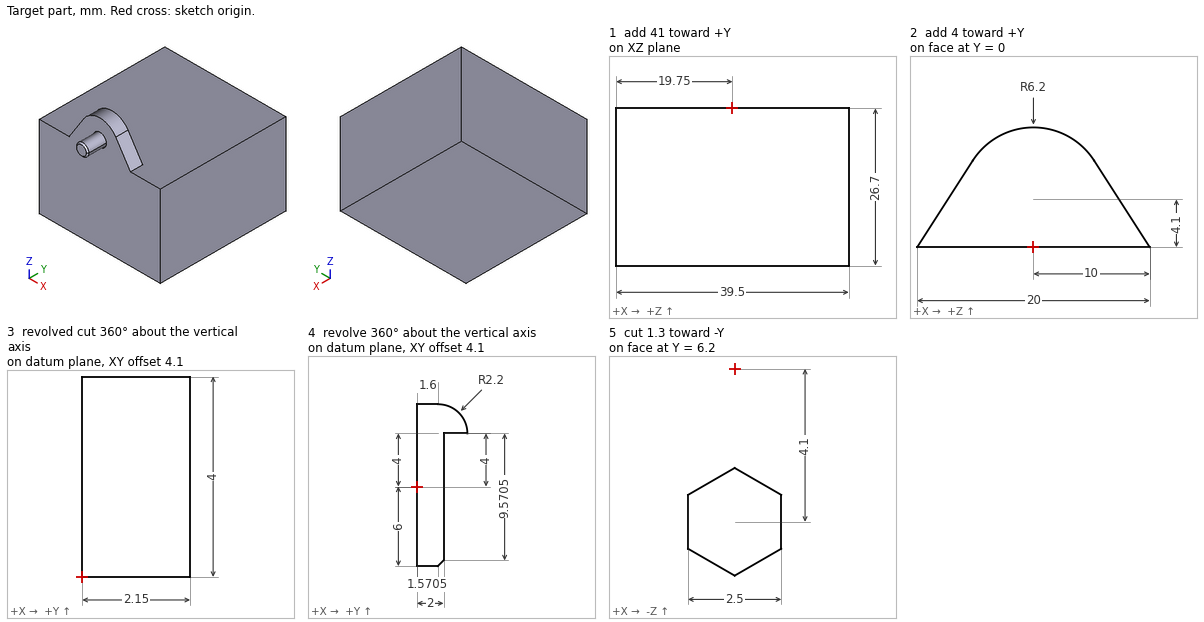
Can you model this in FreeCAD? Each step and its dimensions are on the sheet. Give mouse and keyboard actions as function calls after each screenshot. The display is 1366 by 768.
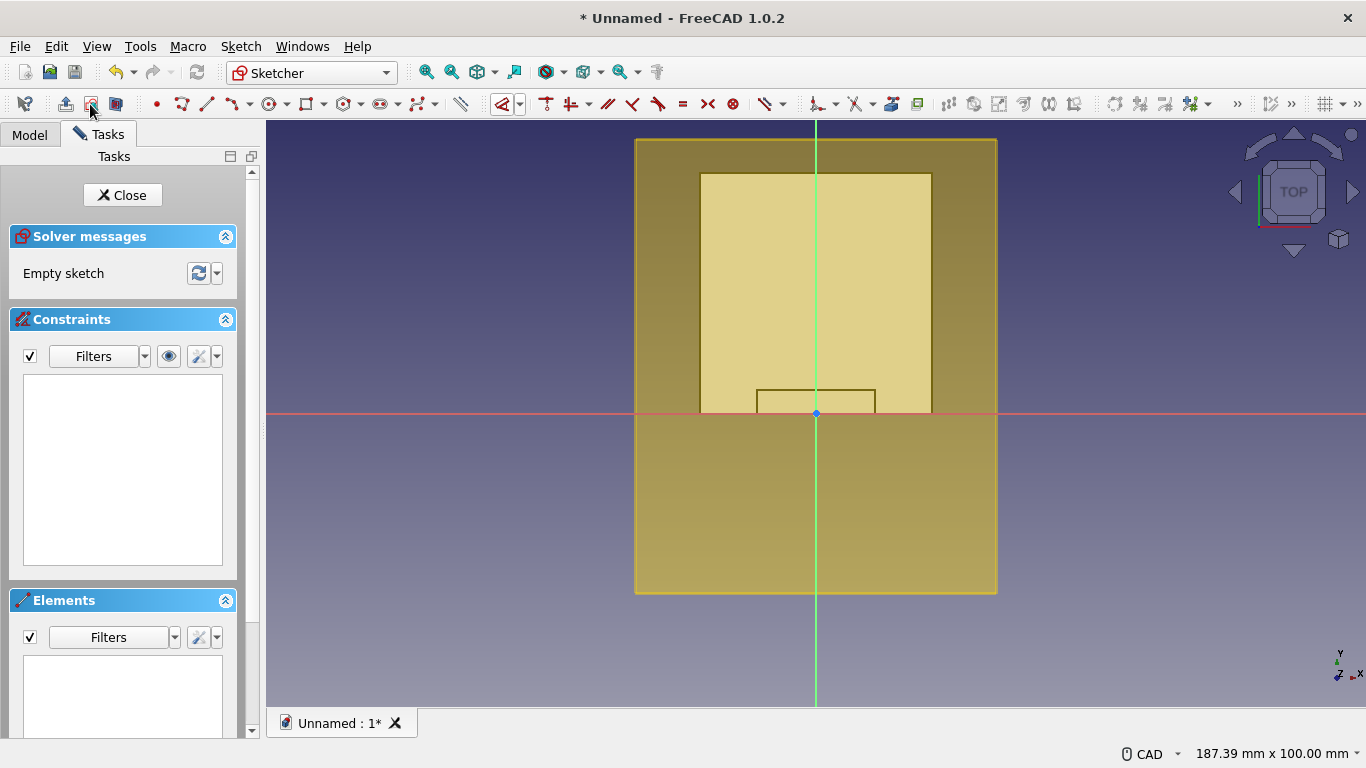
scroll(827, 401, up, 14)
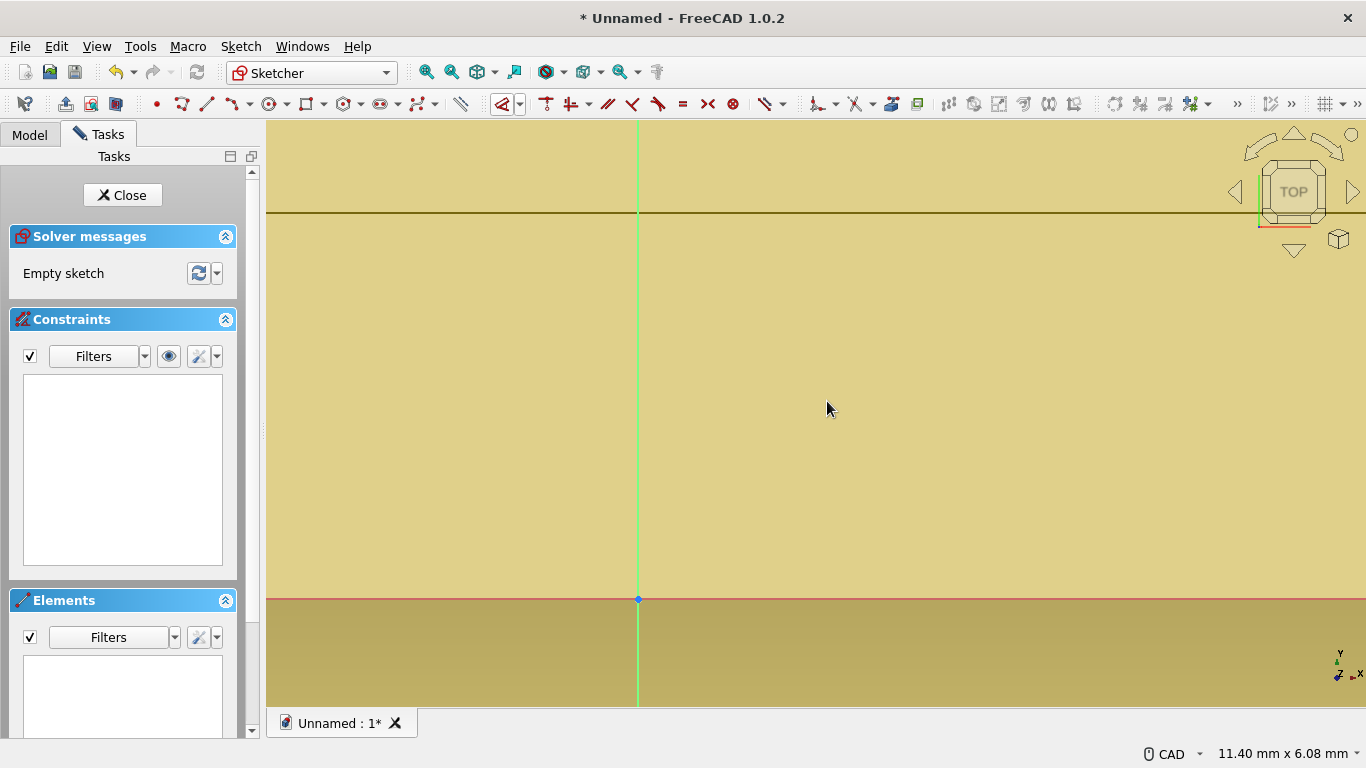
click(306, 104)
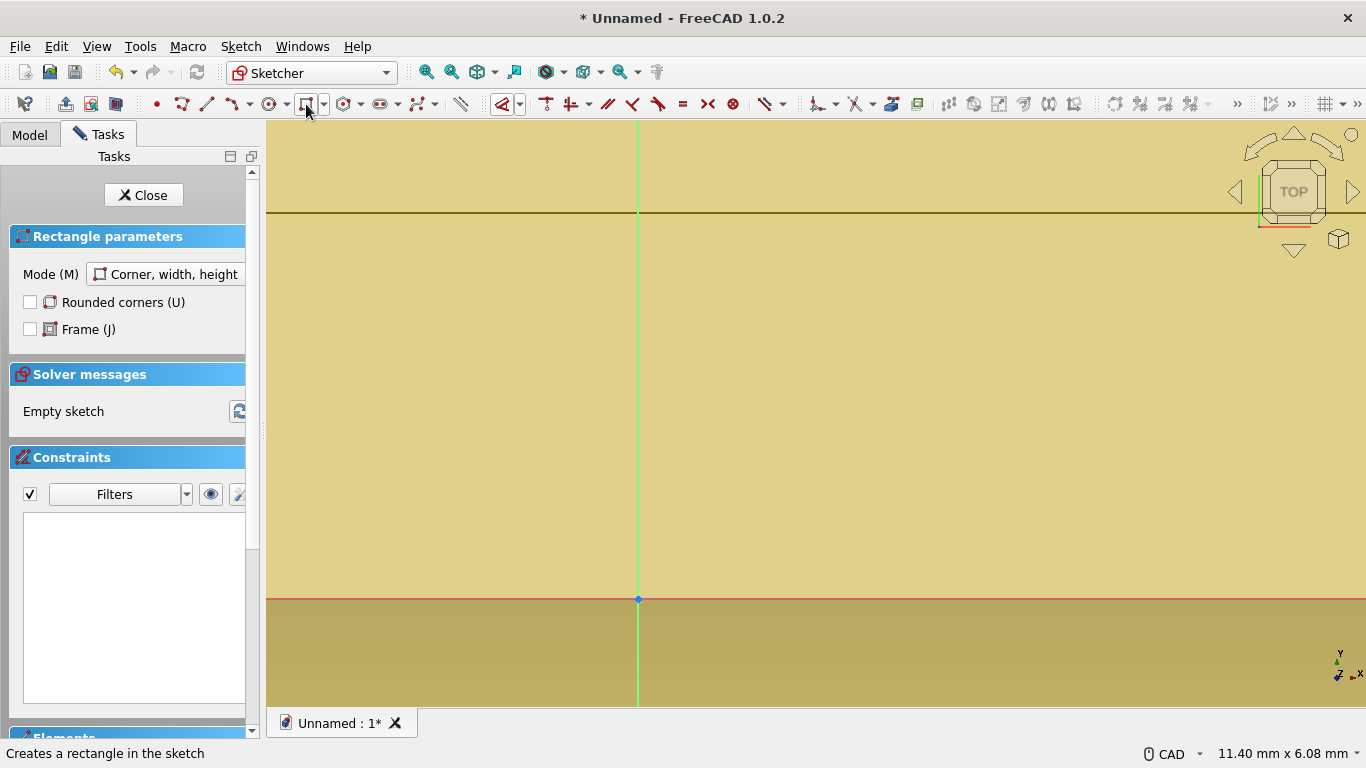
click(638, 599)
move(846, 213)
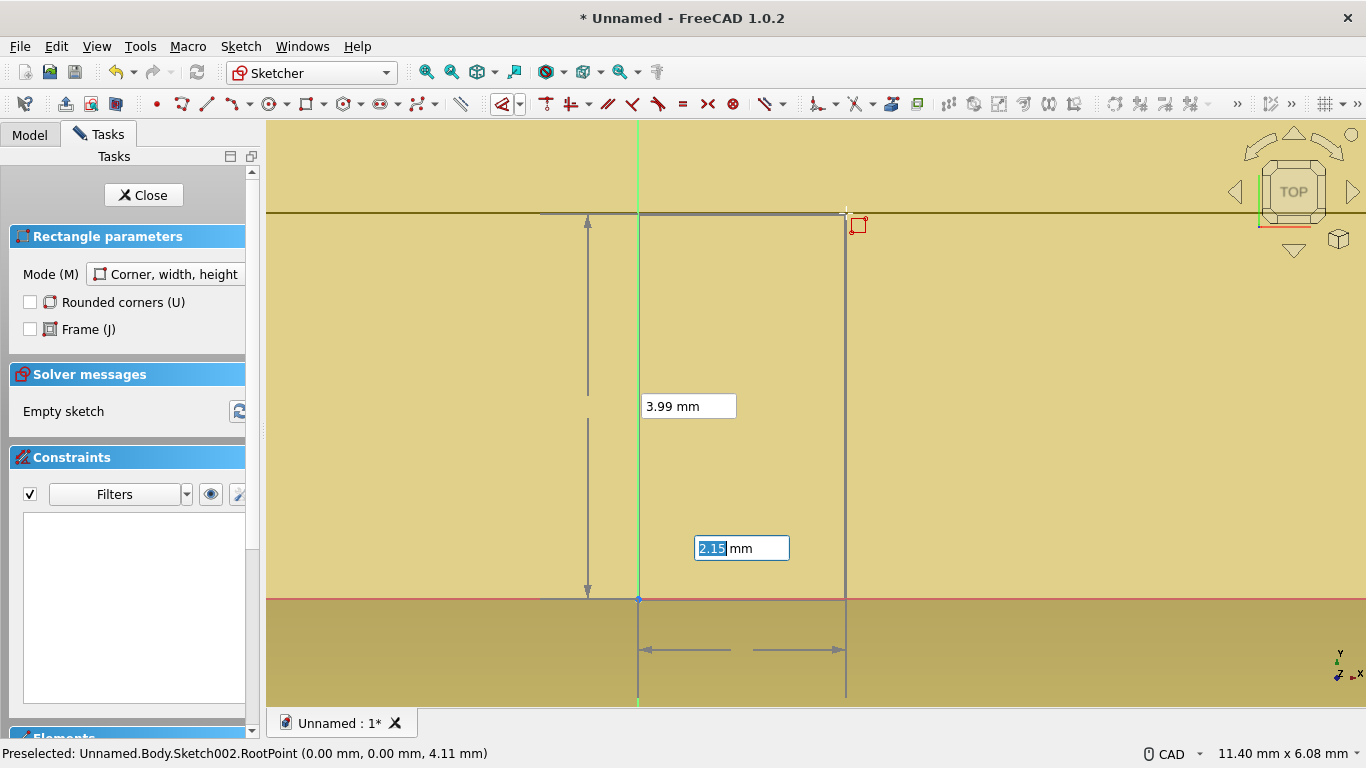
text(2.15)
key(Tab)
text(4)
key(Return)
key(Escape)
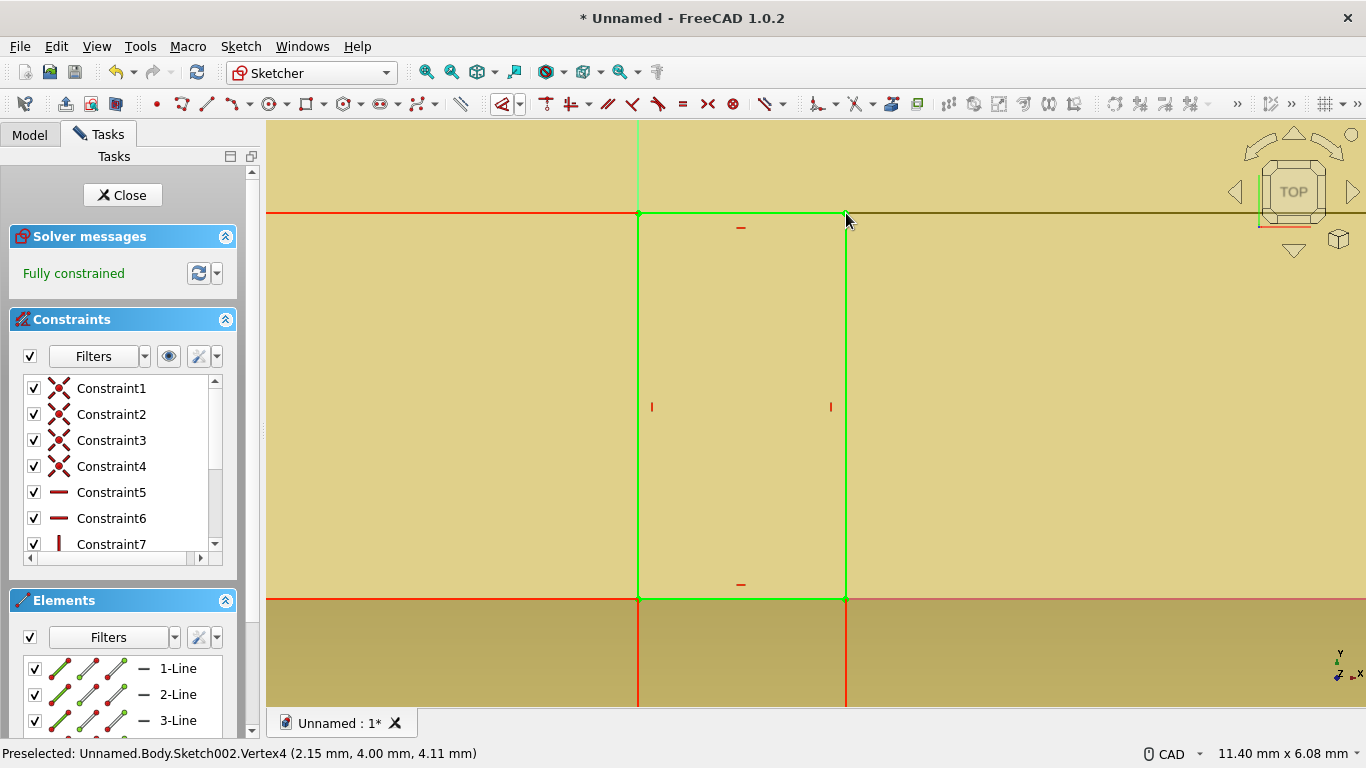
click(123, 195)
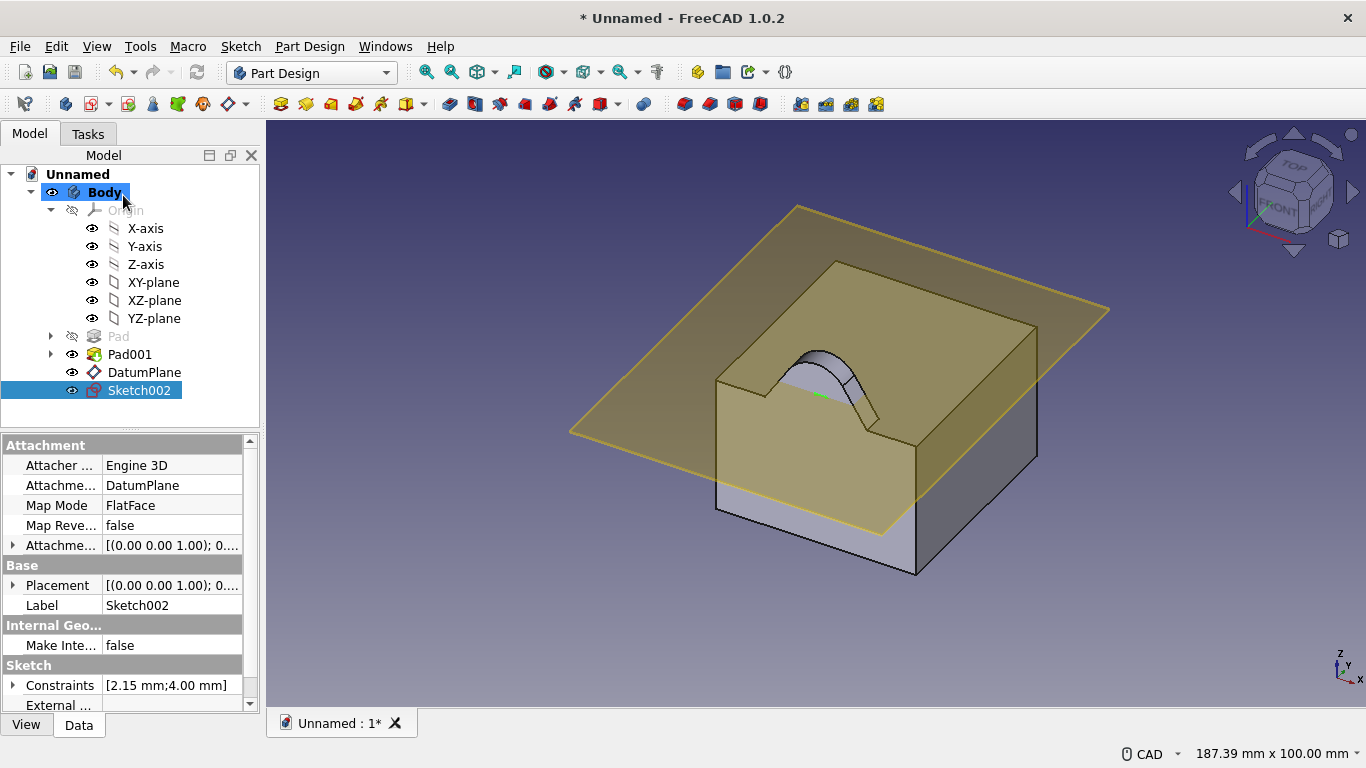
click(500, 104)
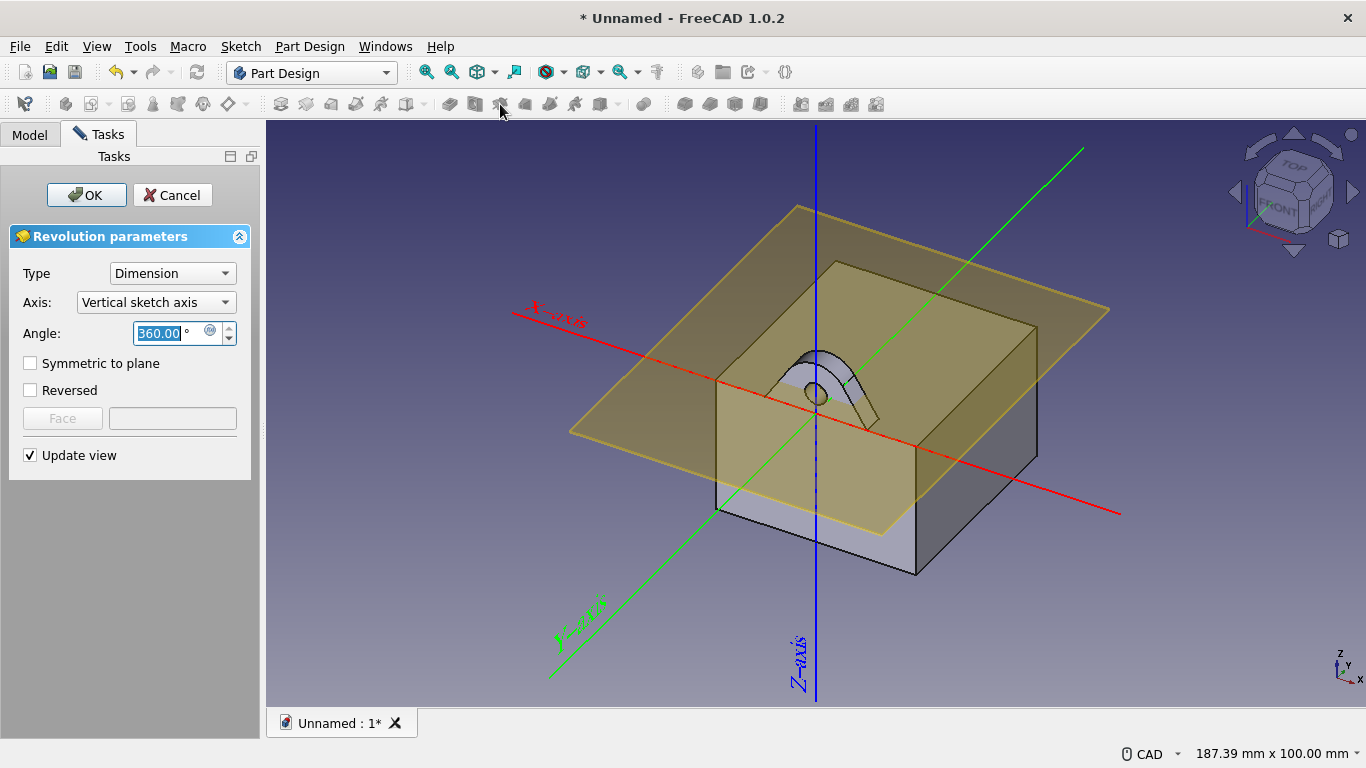
click(87, 195)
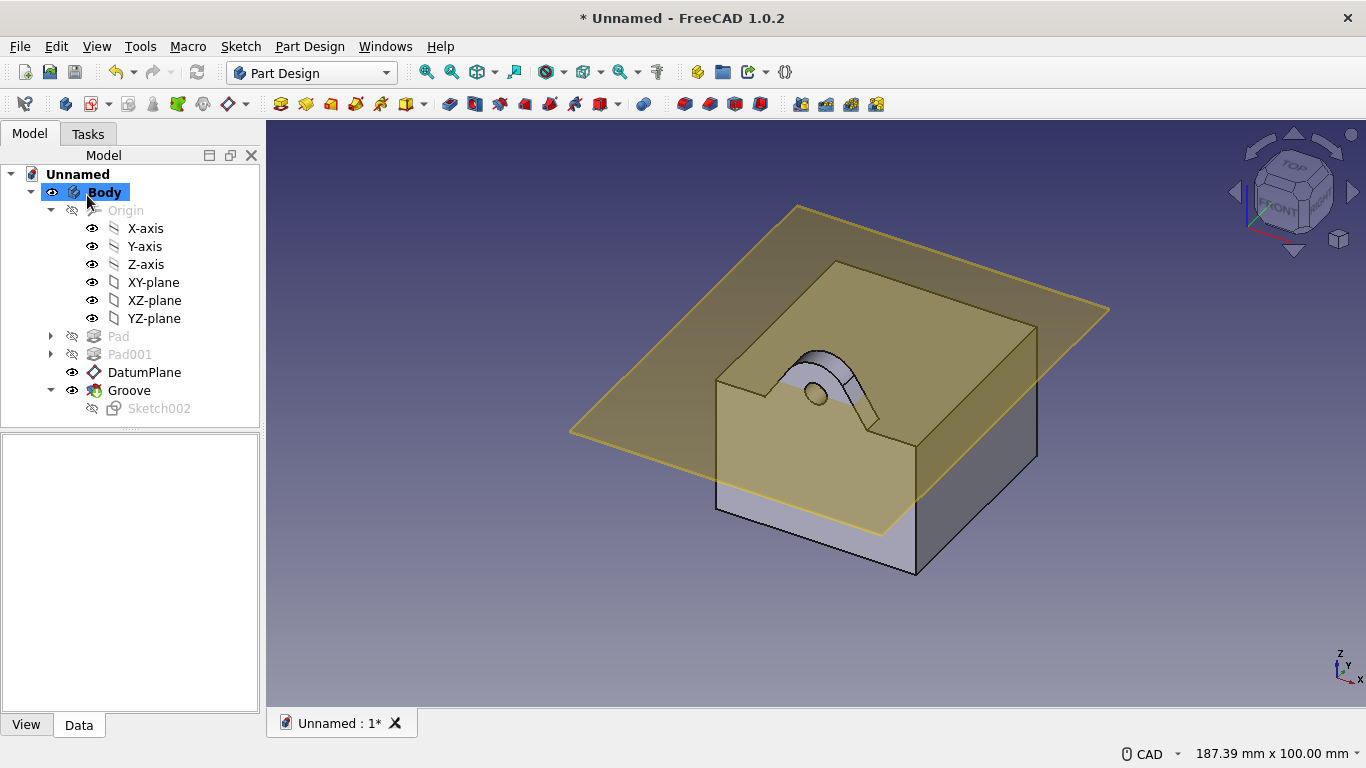
click(117, 372)
key(space)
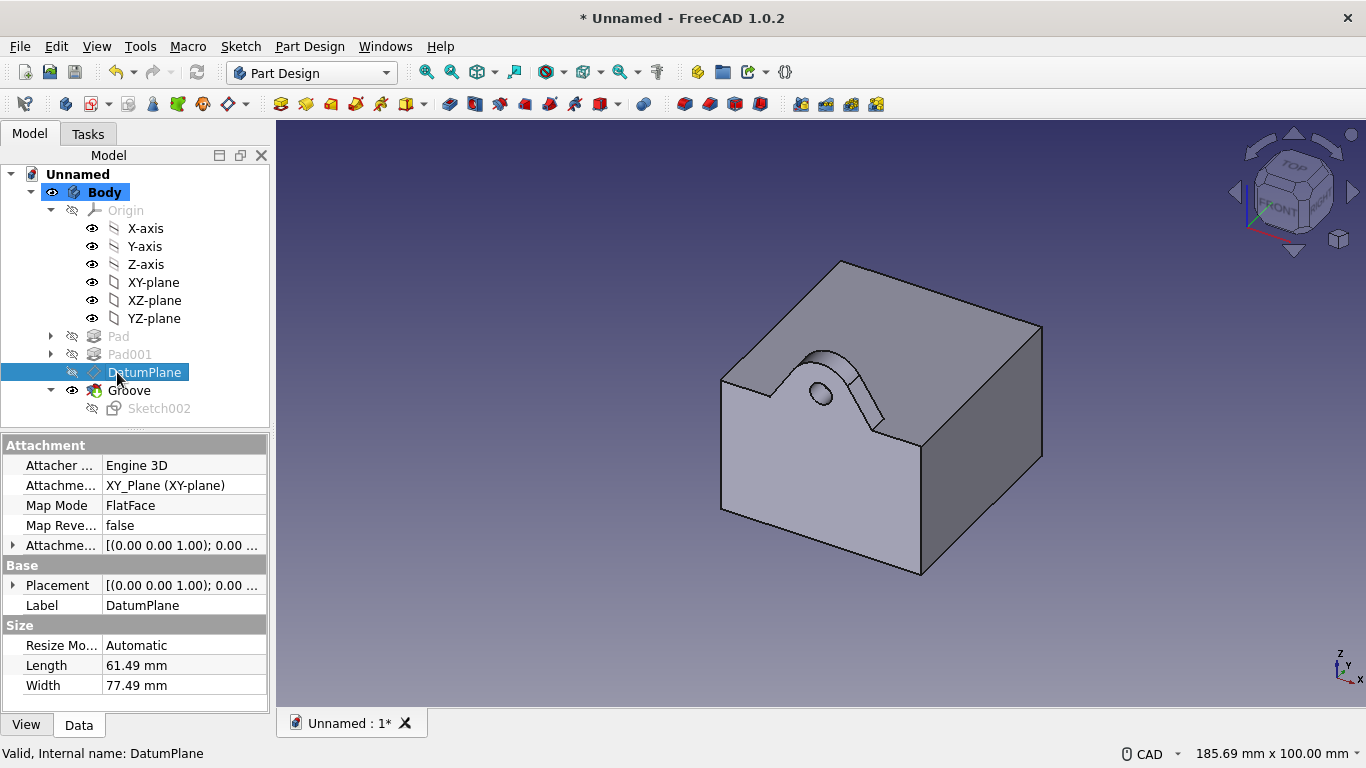
click(137, 282)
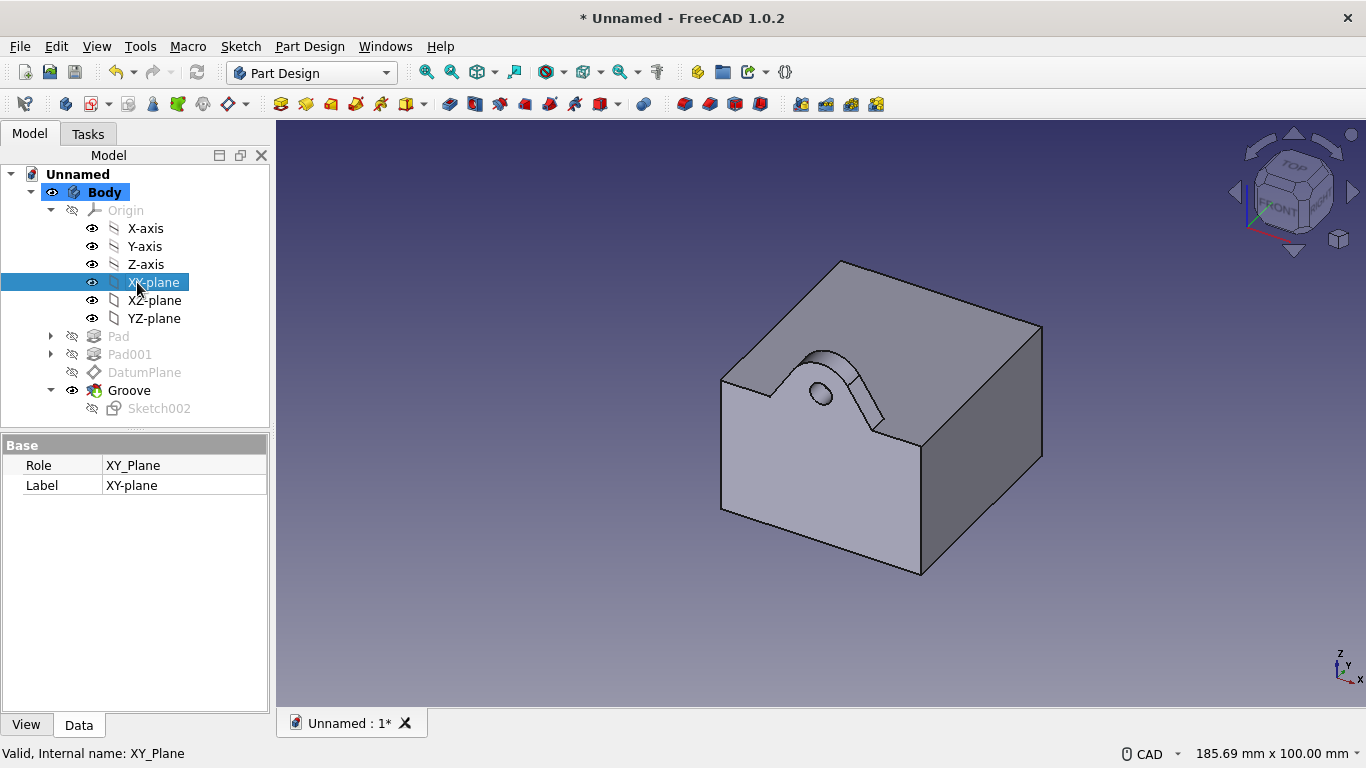
click(228, 104)